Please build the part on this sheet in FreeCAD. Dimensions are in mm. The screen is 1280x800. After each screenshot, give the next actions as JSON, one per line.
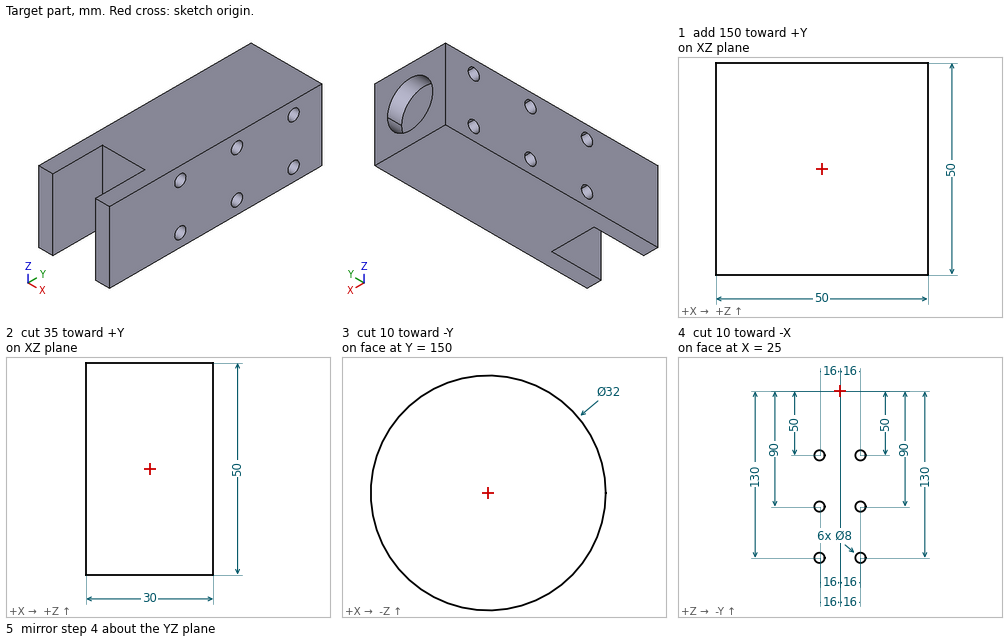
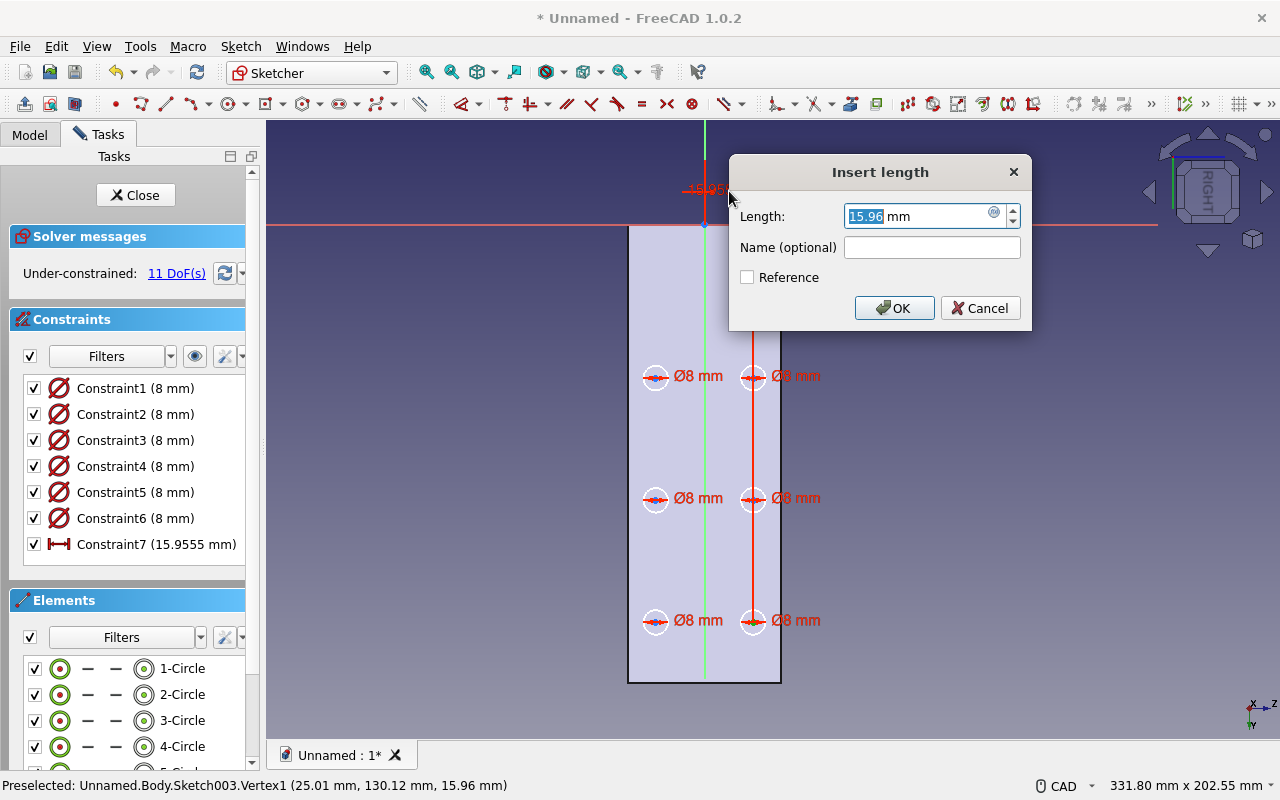
{"action": "type", "text": "16"}
{"action": "key", "text": "Return"}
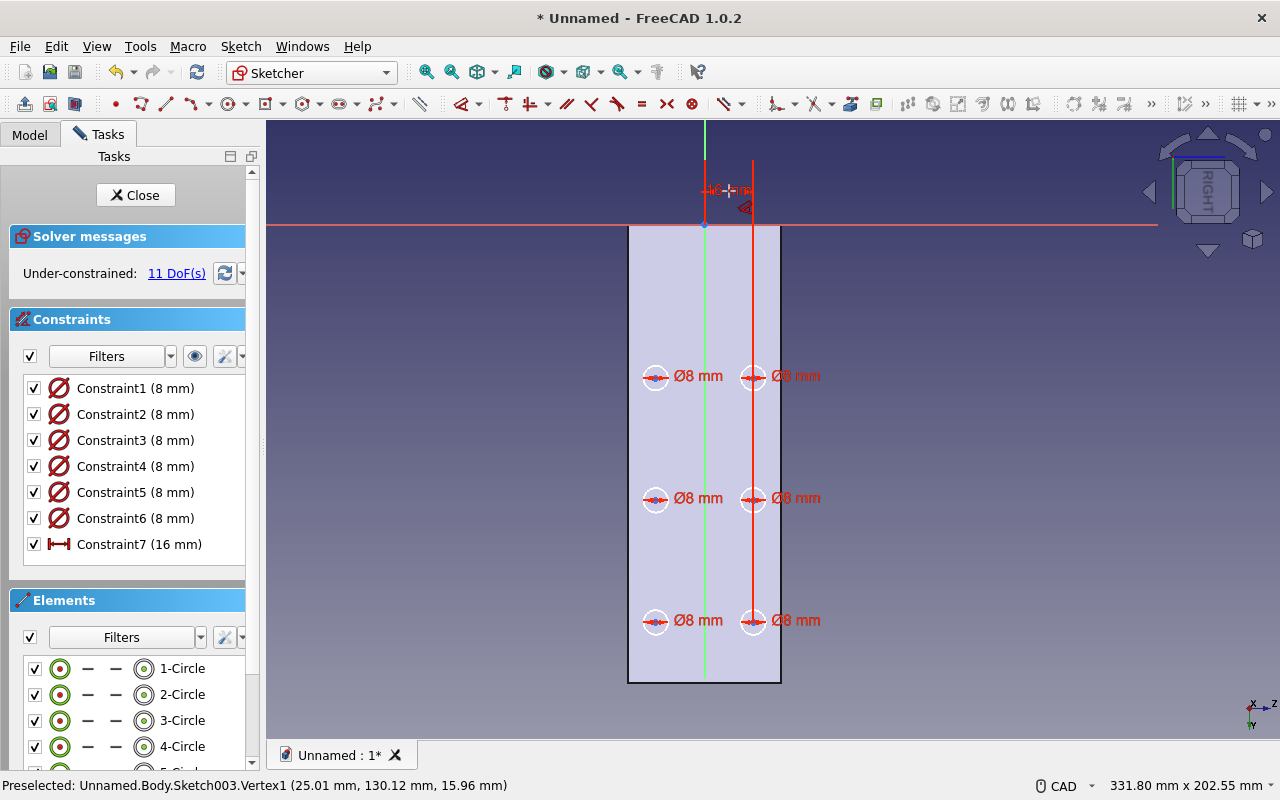
{"action": "left_click", "coordinate": [656, 622]}
{"action": "left_click", "coordinate": [680, 656]}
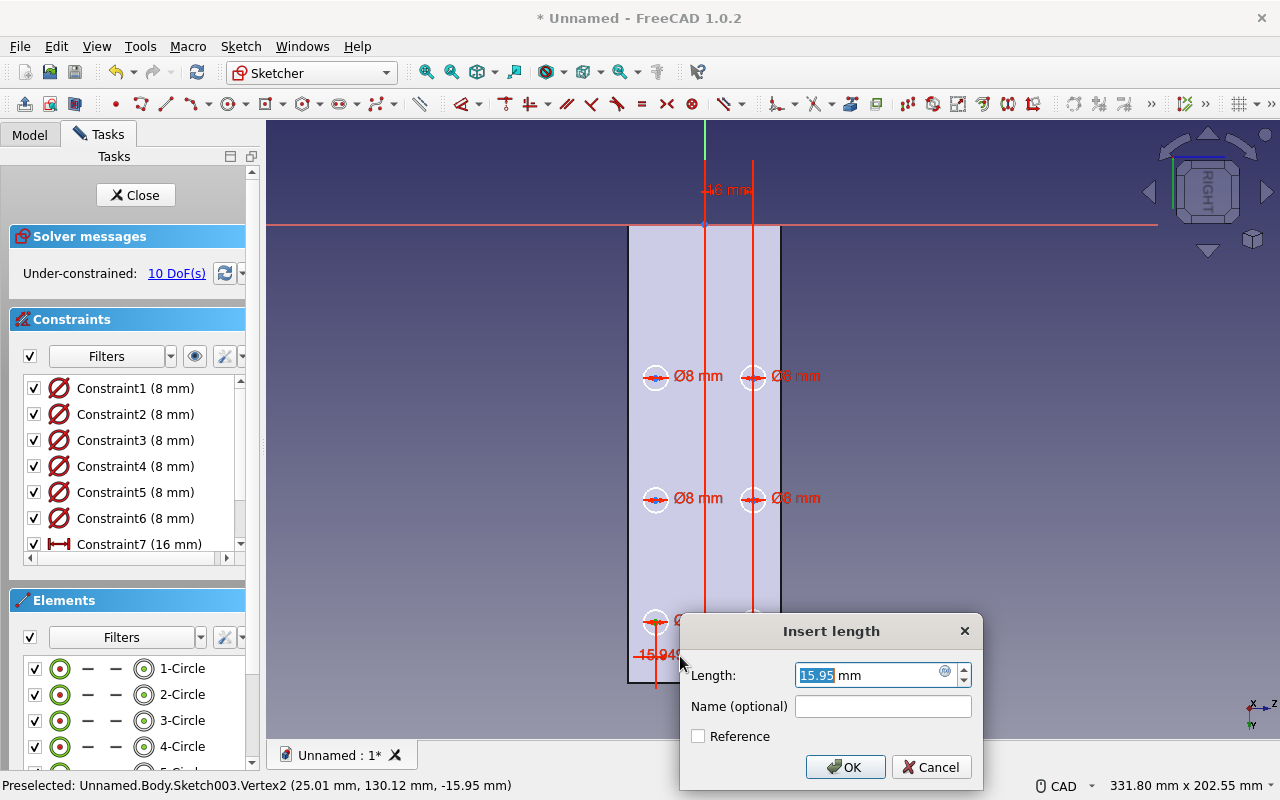
{"action": "type", "text": "16"}
{"action": "key", "text": "Return"}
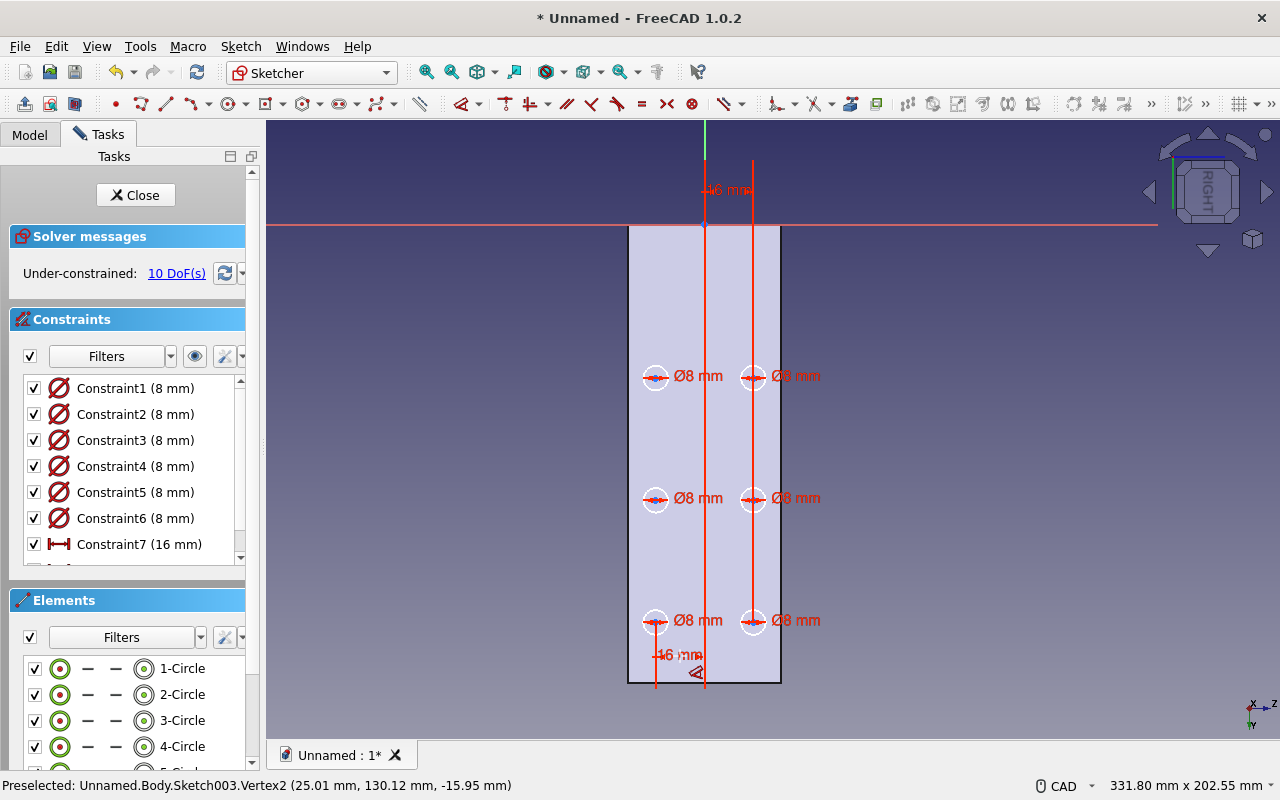
{"action": "left_click", "coordinate": [753, 500]}
{"action": "left_click", "coordinate": [729, 534]}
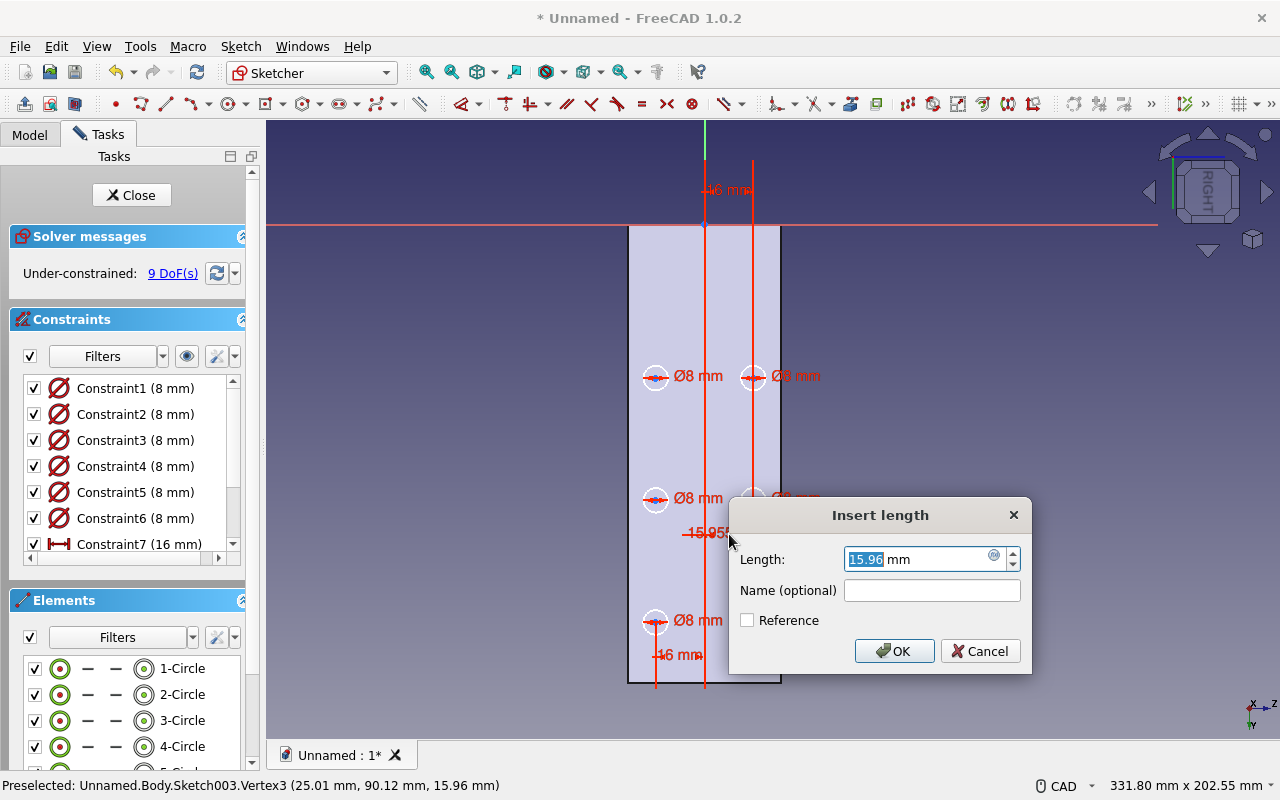
{"action": "type", "text": "16"}
{"action": "key", "text": "Return"}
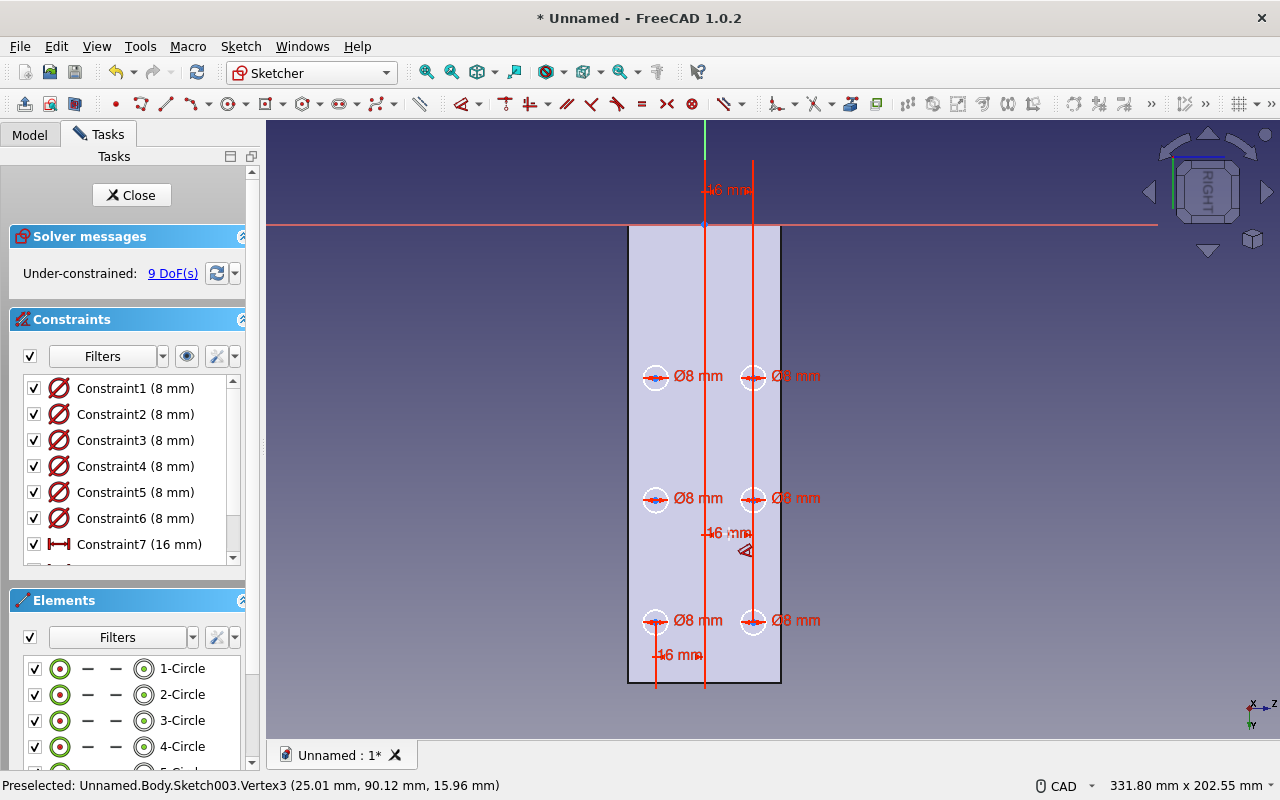
{"action": "left_click", "coordinate": [753, 500]}
{"action": "left_click", "coordinate": [787, 363]}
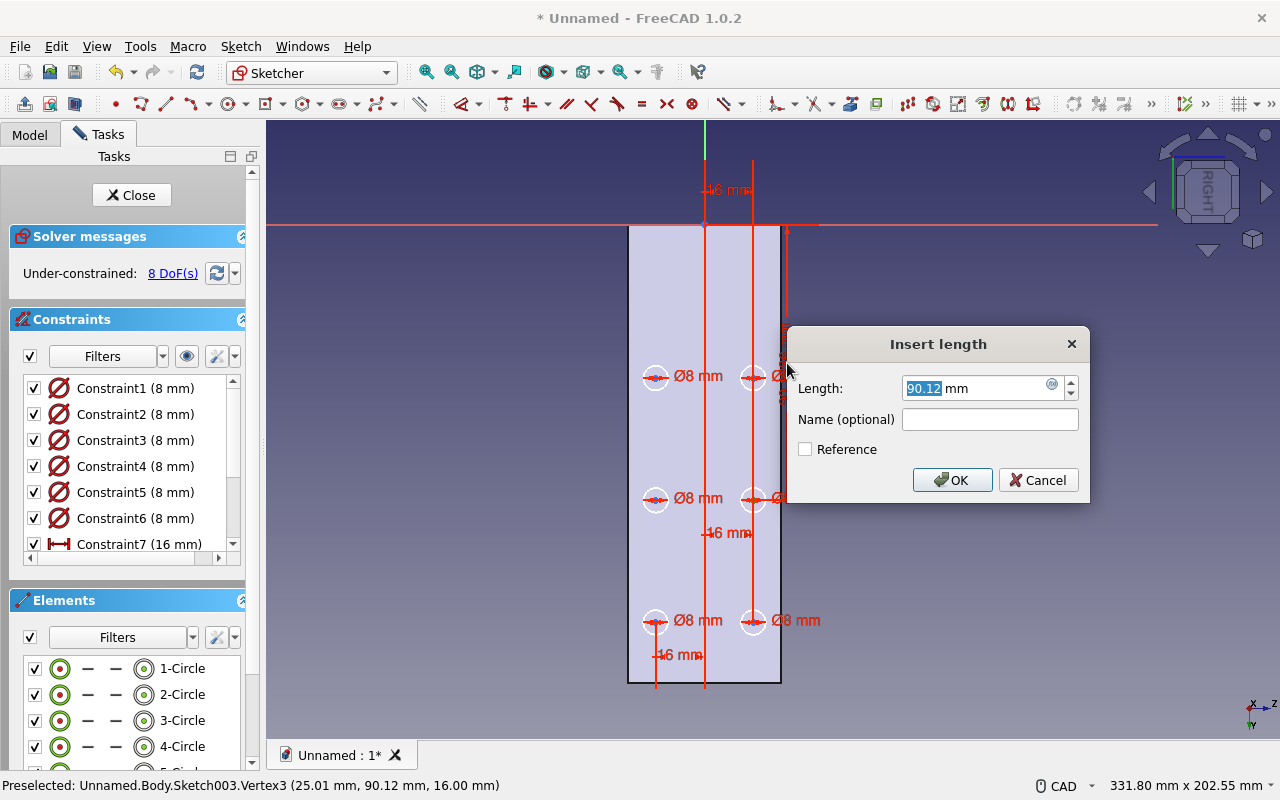
{"action": "type", "text": "90"}
{"action": "key", "text": "Return"}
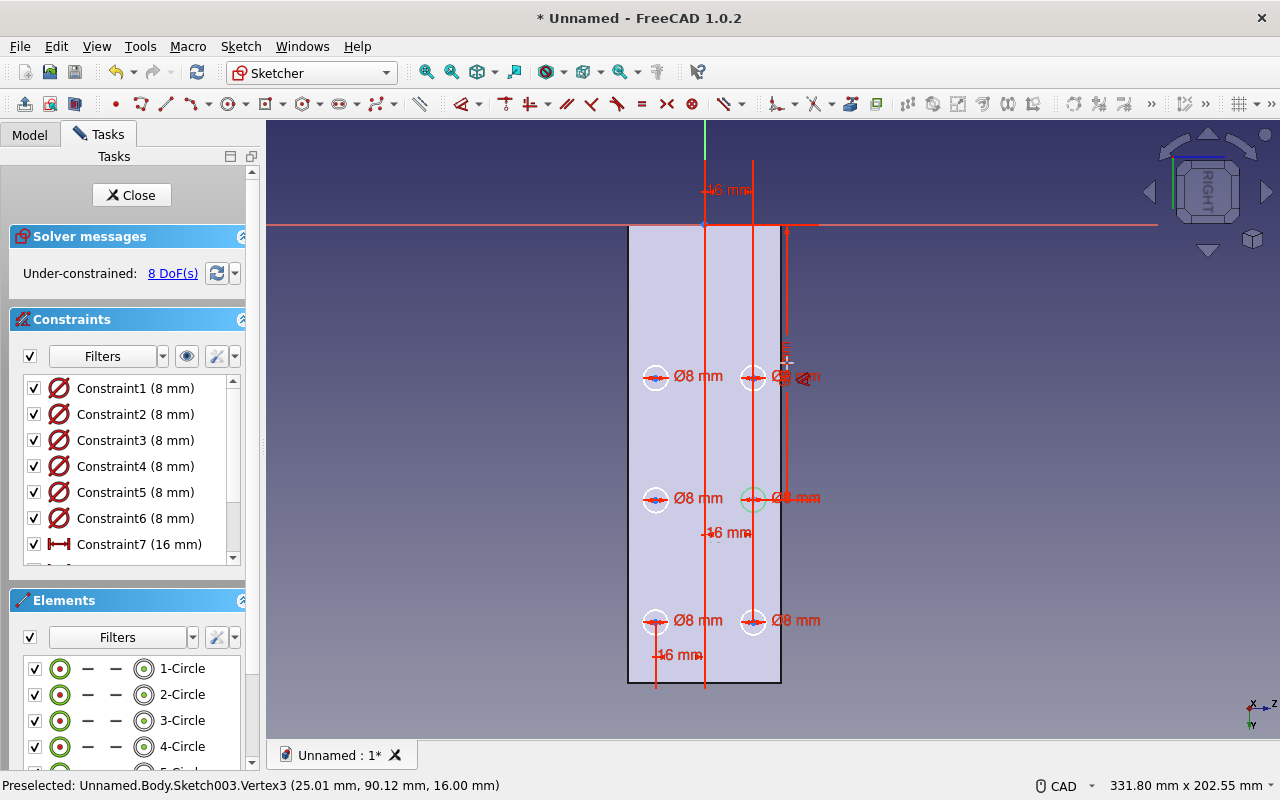
{"action": "left_click", "coordinate": [753, 378]}
{"action": "left_click", "coordinate": [729, 412]}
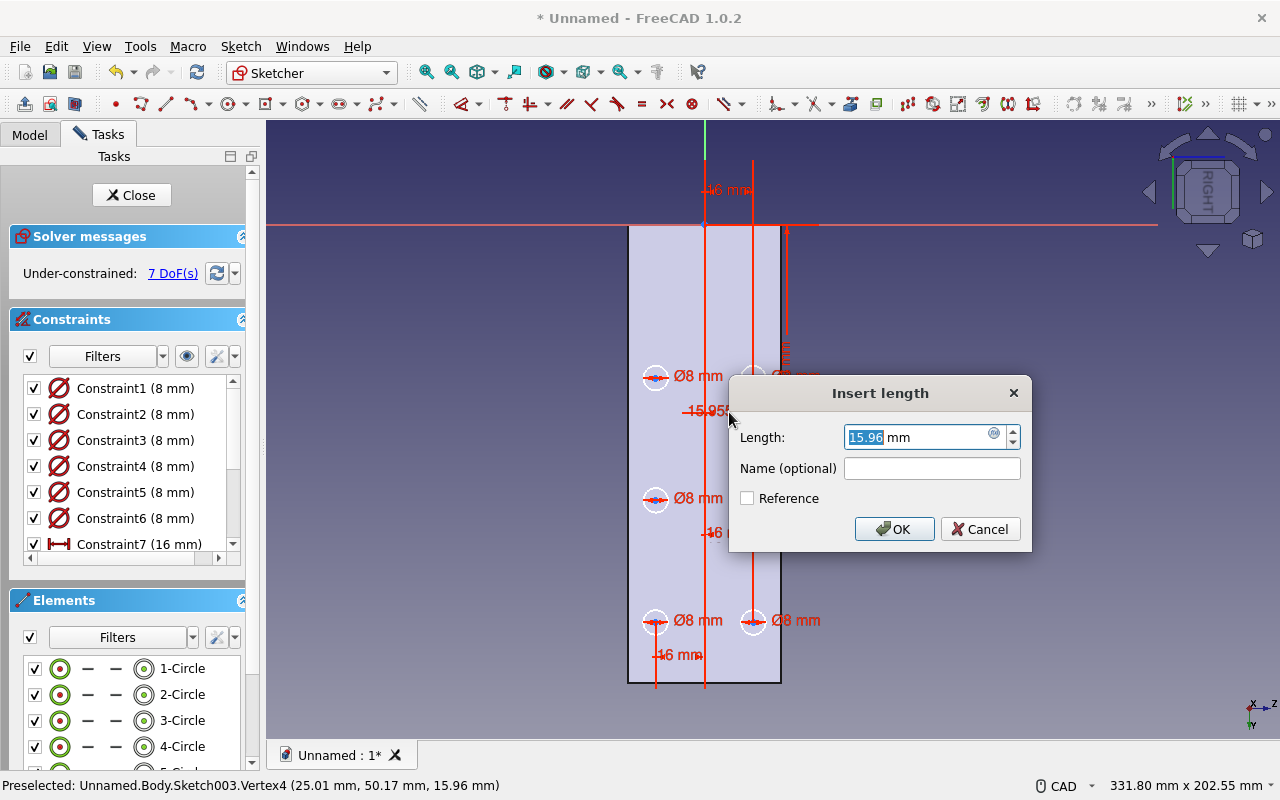
{"action": "type", "text": "16"}
{"action": "key", "text": "Return"}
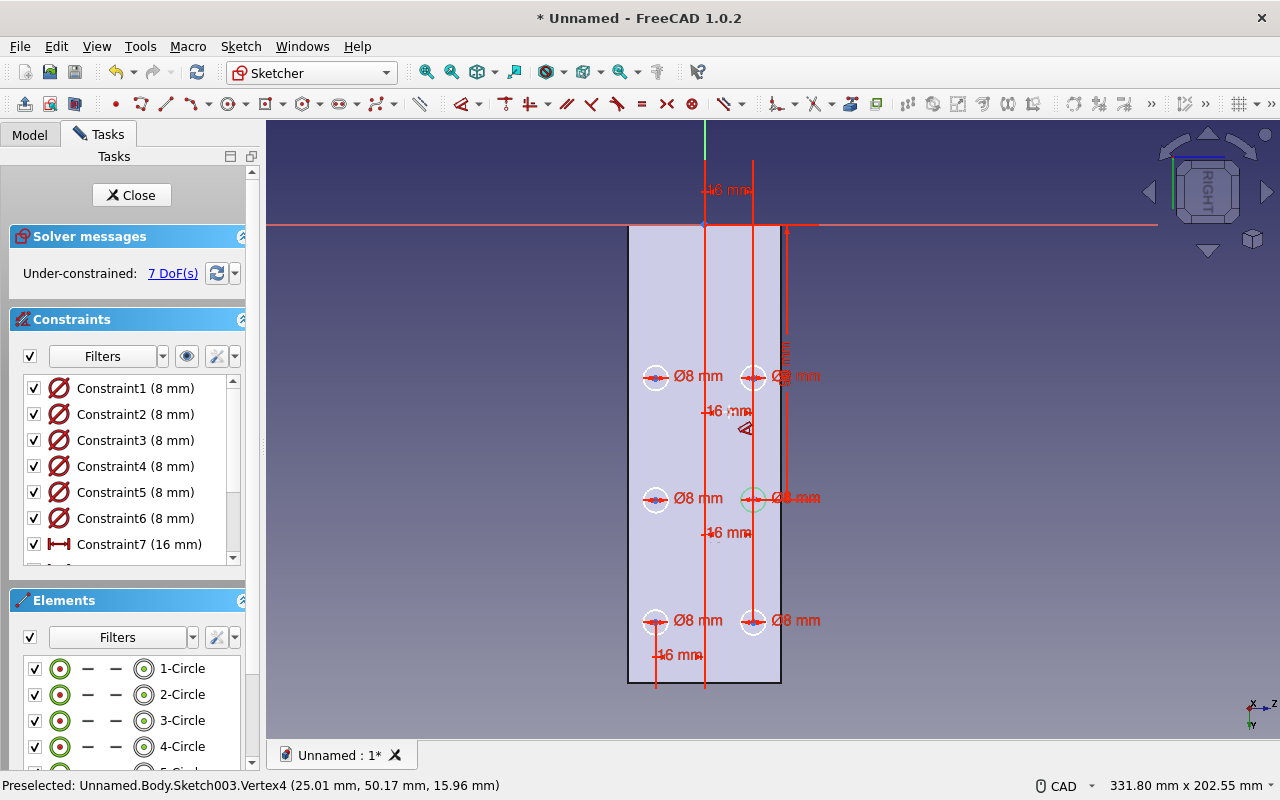
{"action": "left_click", "coordinate": [753, 378]}
{"action": "left_click", "coordinate": [787, 301]}